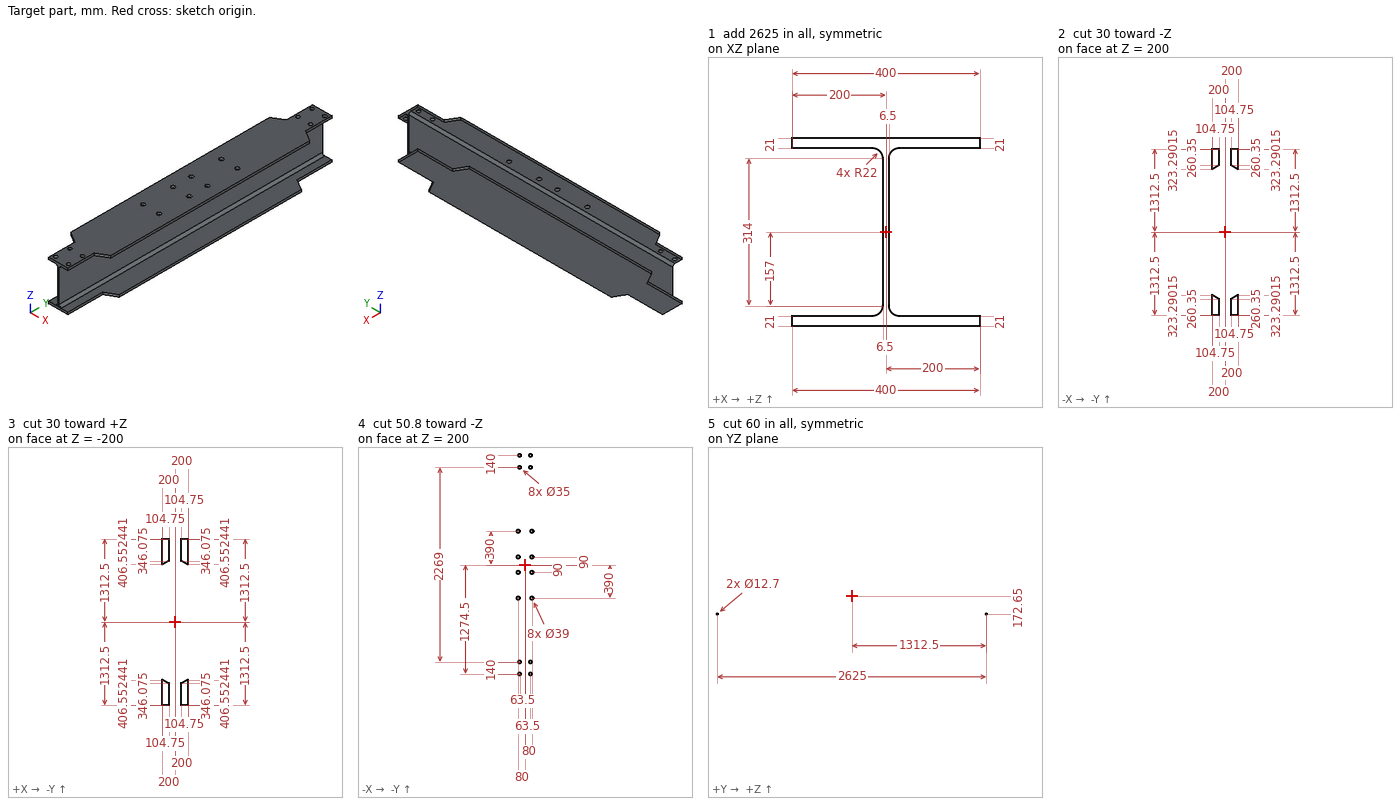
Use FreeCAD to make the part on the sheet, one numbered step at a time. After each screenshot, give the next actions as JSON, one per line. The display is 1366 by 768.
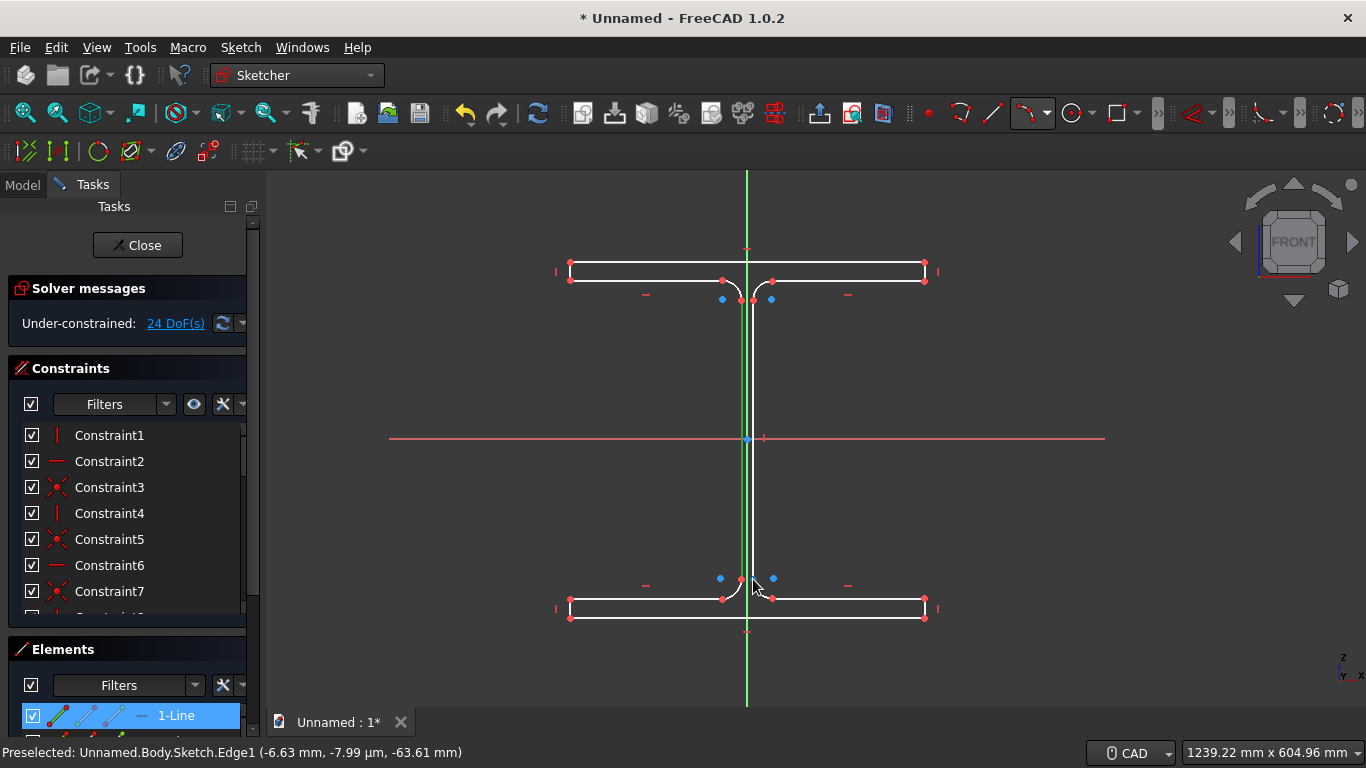
{"action": "scroll", "coordinate": [740, 291], "scroll_direction": "up", "scroll_amount": 3}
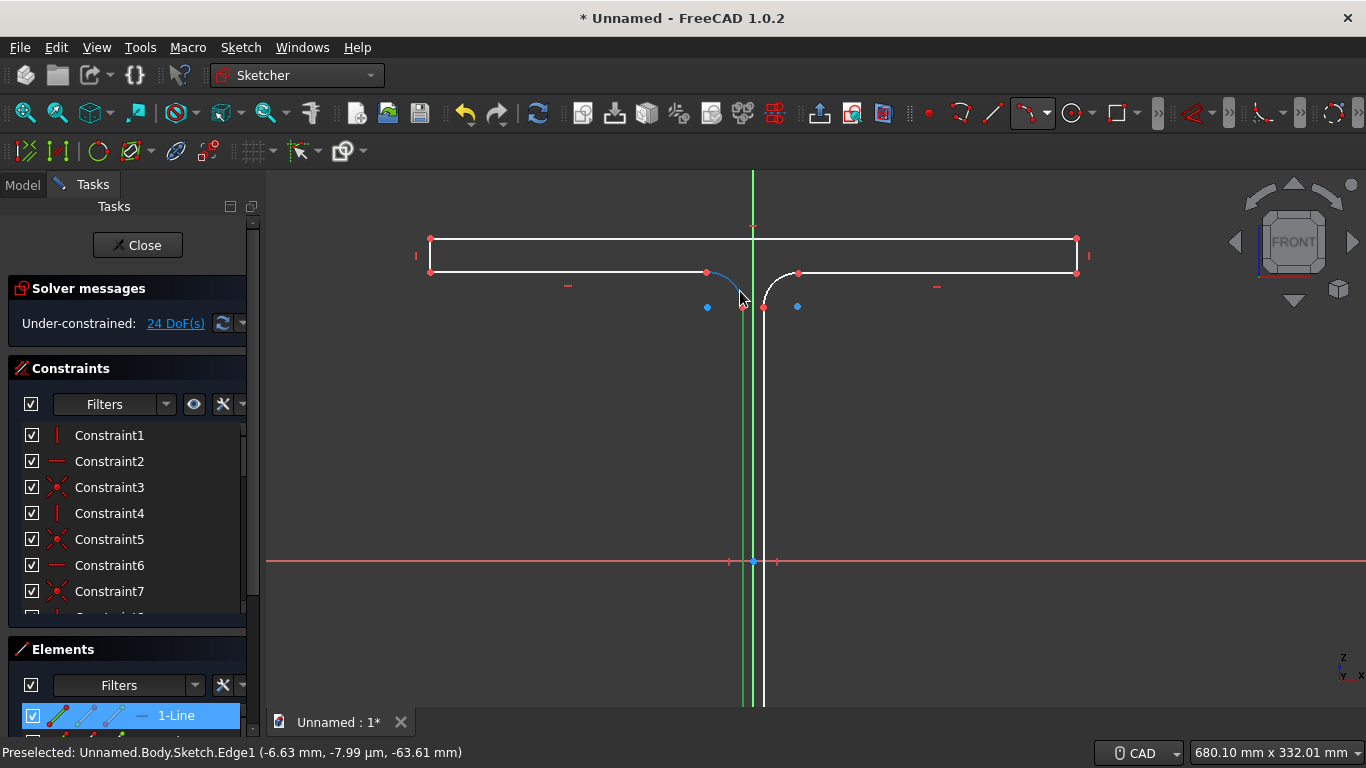
{"action": "left_click", "coordinate": [739, 291]}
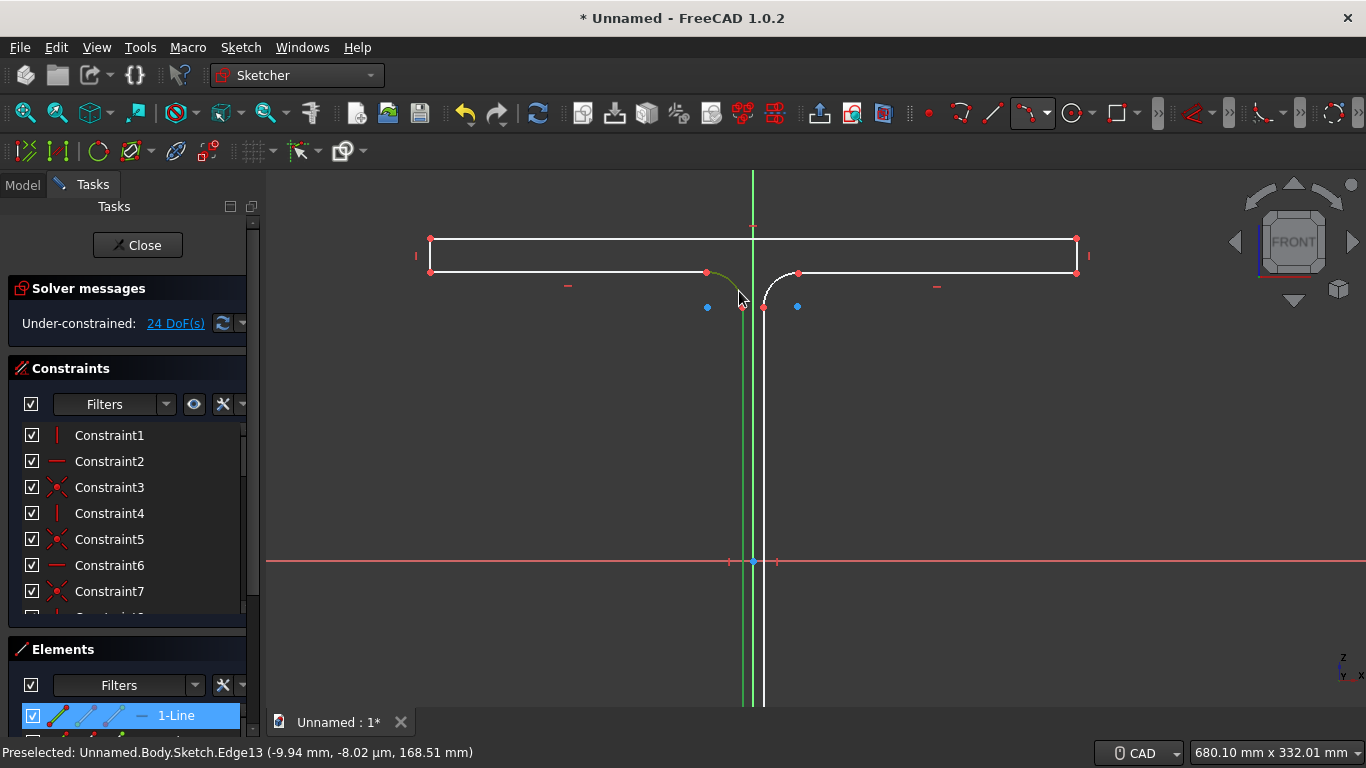
{"action": "key", "text": "t"}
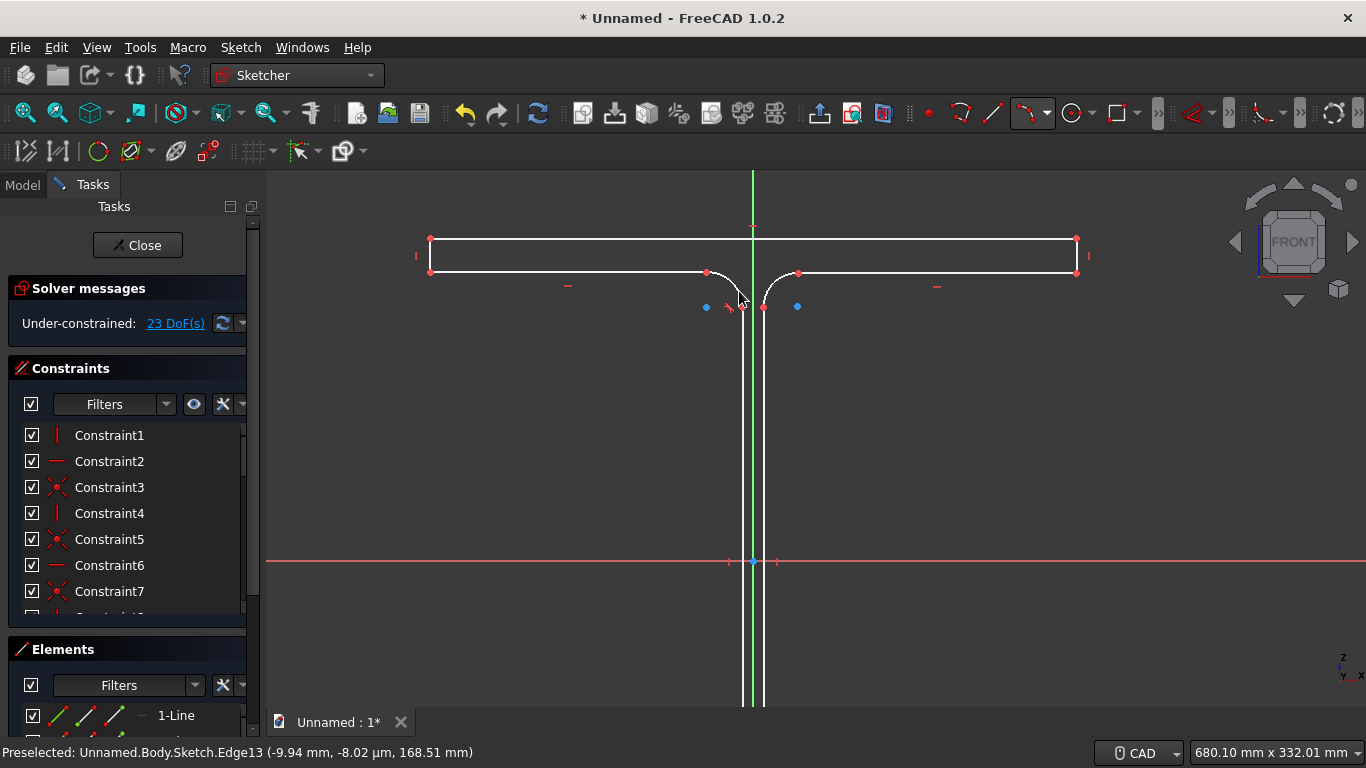
{"action": "scroll", "coordinate": [743, 663], "scroll_direction": "up", "scroll_amount": 2}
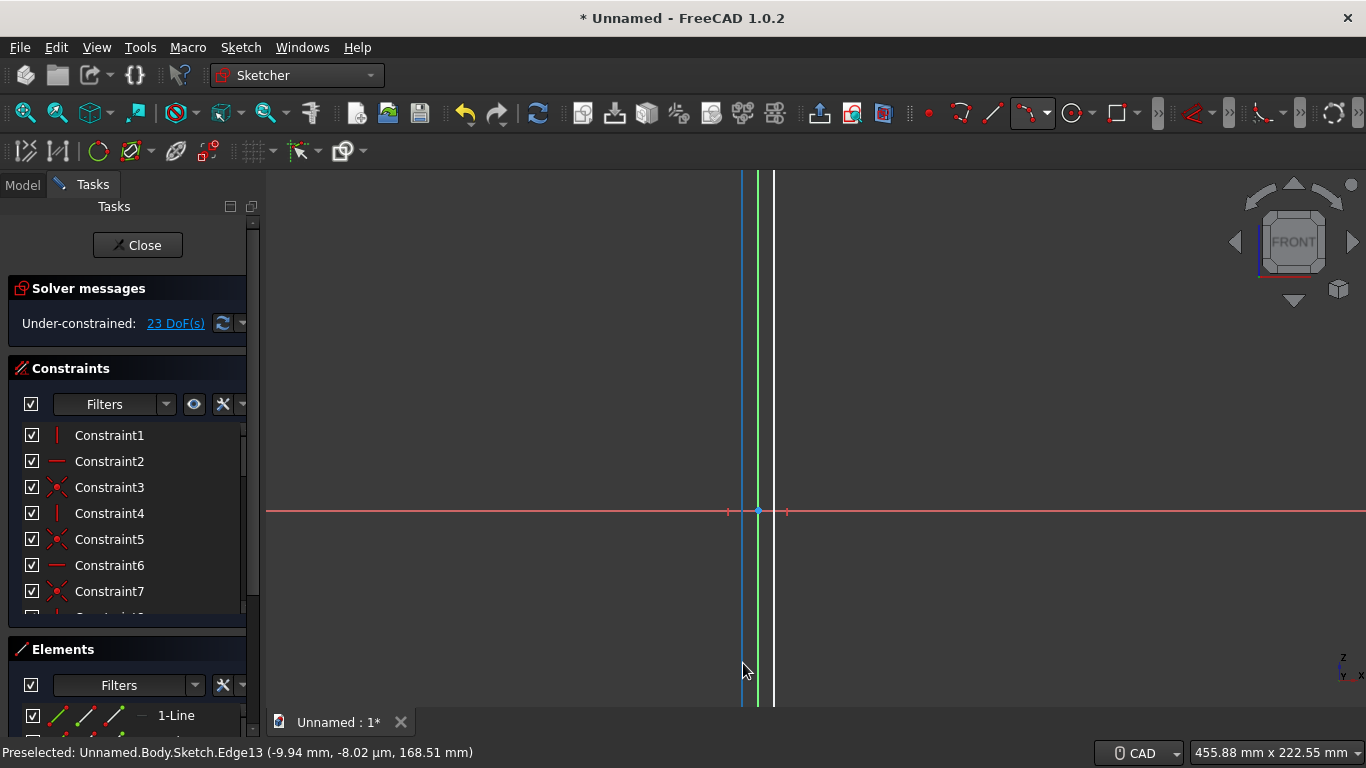
{"action": "left_click", "coordinate": [742, 663]}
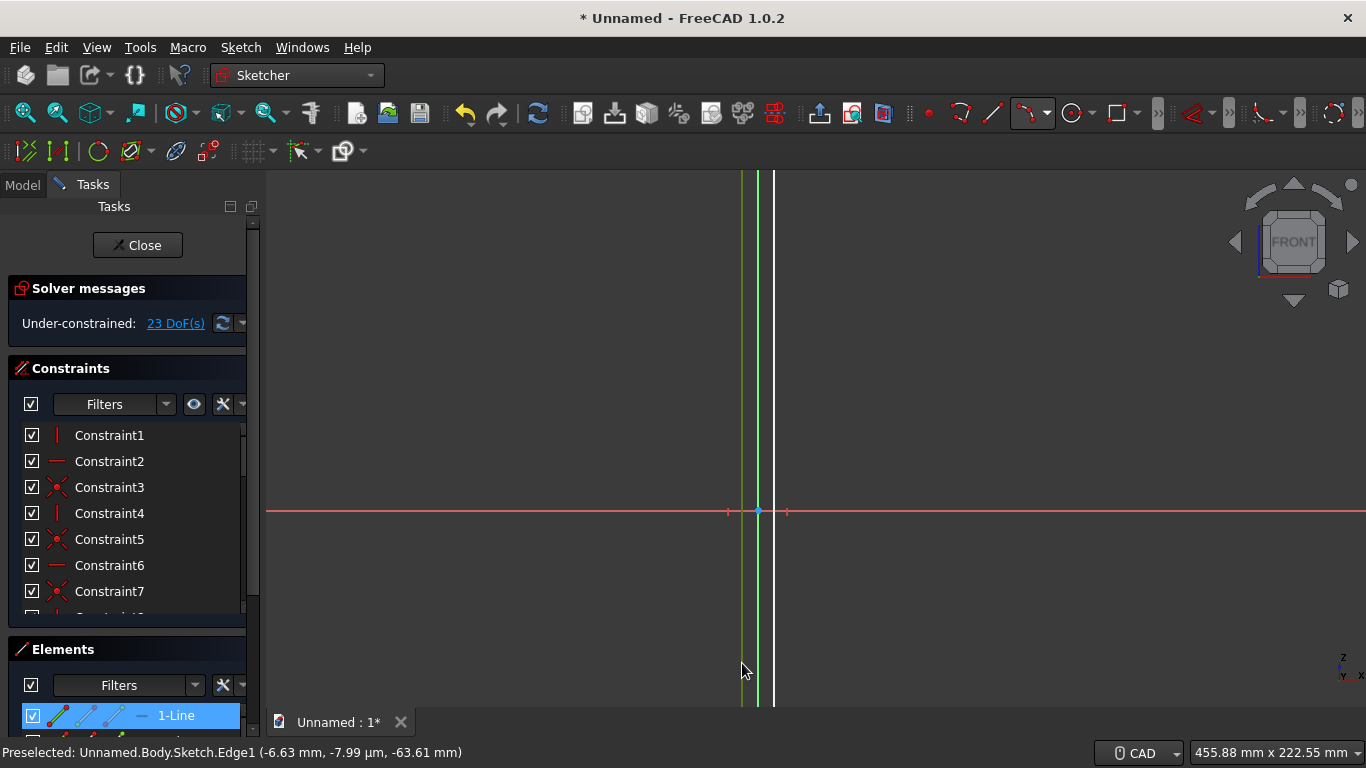
{"action": "scroll", "coordinate": [741, 397], "scroll_direction": "down", "scroll_amount": 5}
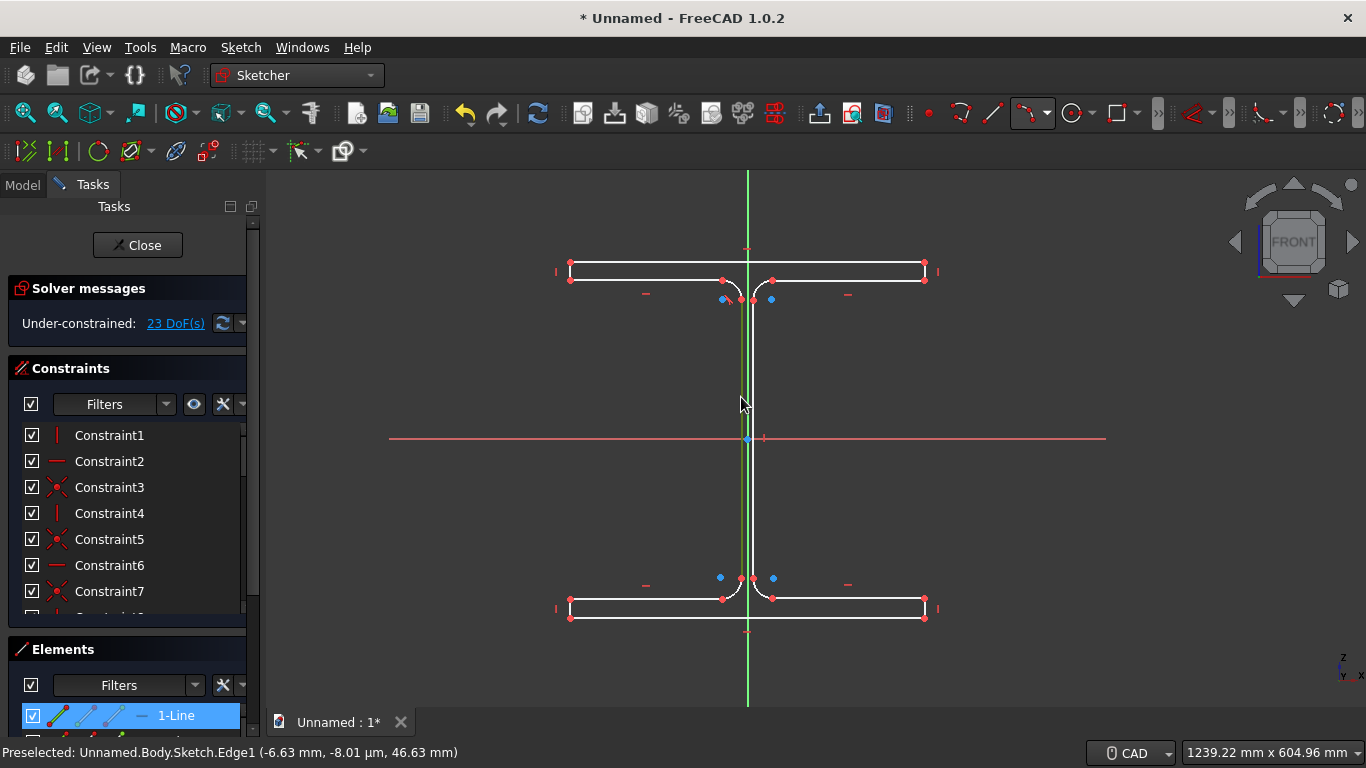
{"action": "scroll", "coordinate": [731, 596], "scroll_direction": "up", "scroll_amount": 3}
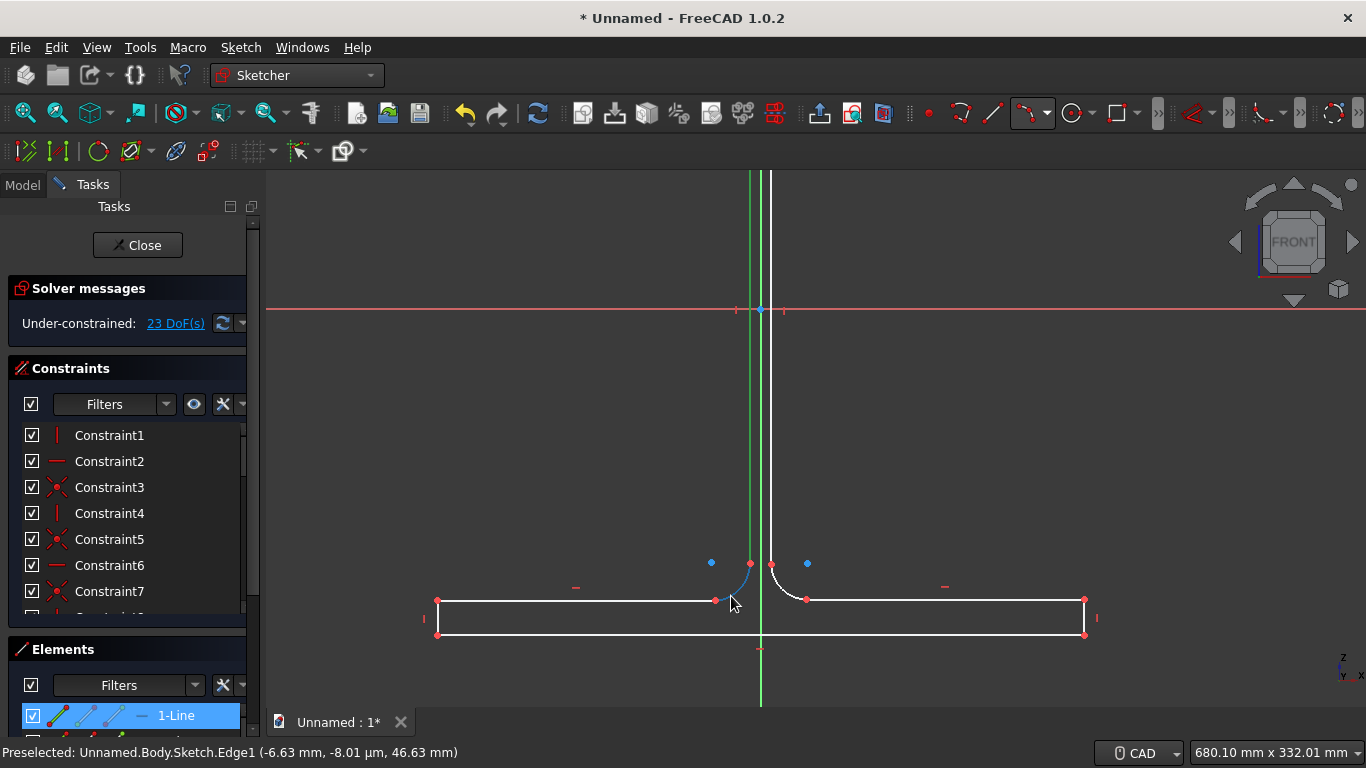
{"action": "left_click", "coordinate": [731, 596]}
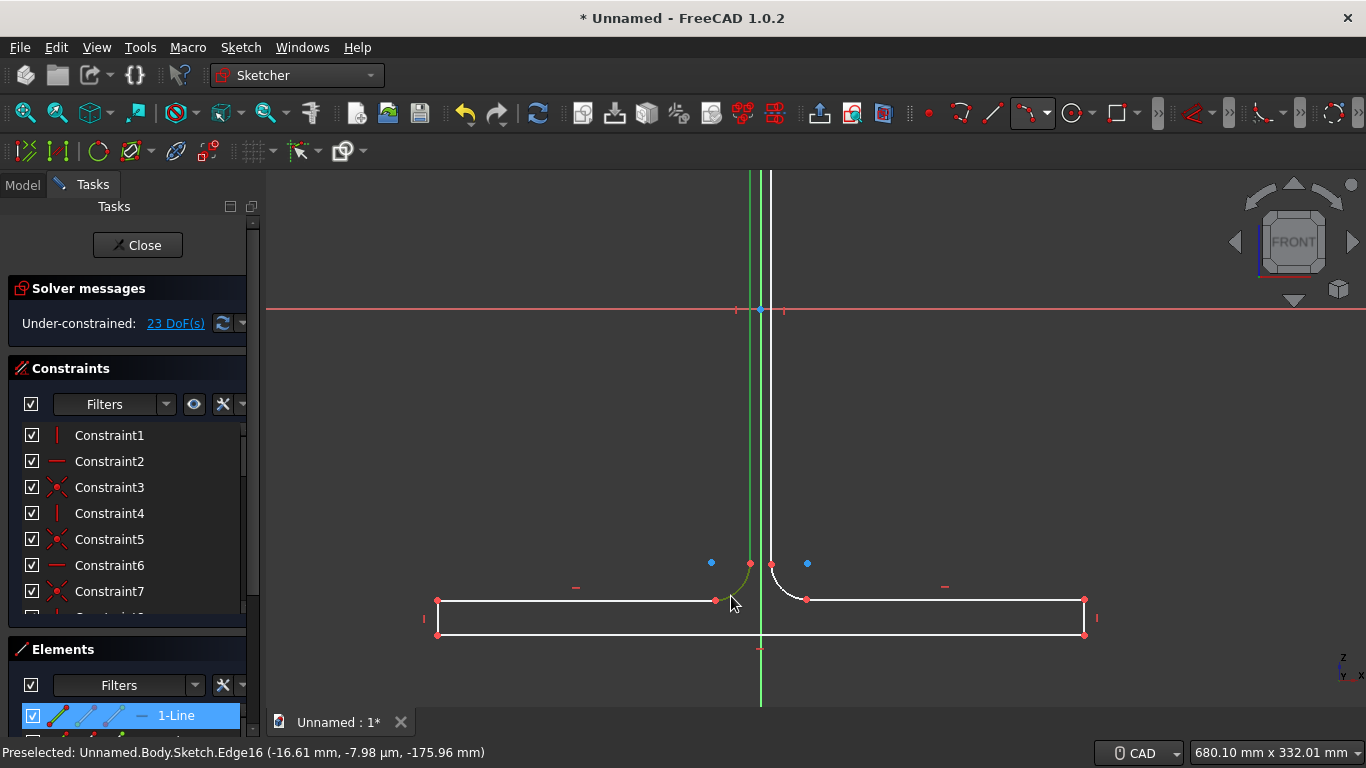
{"action": "key", "text": "t"}